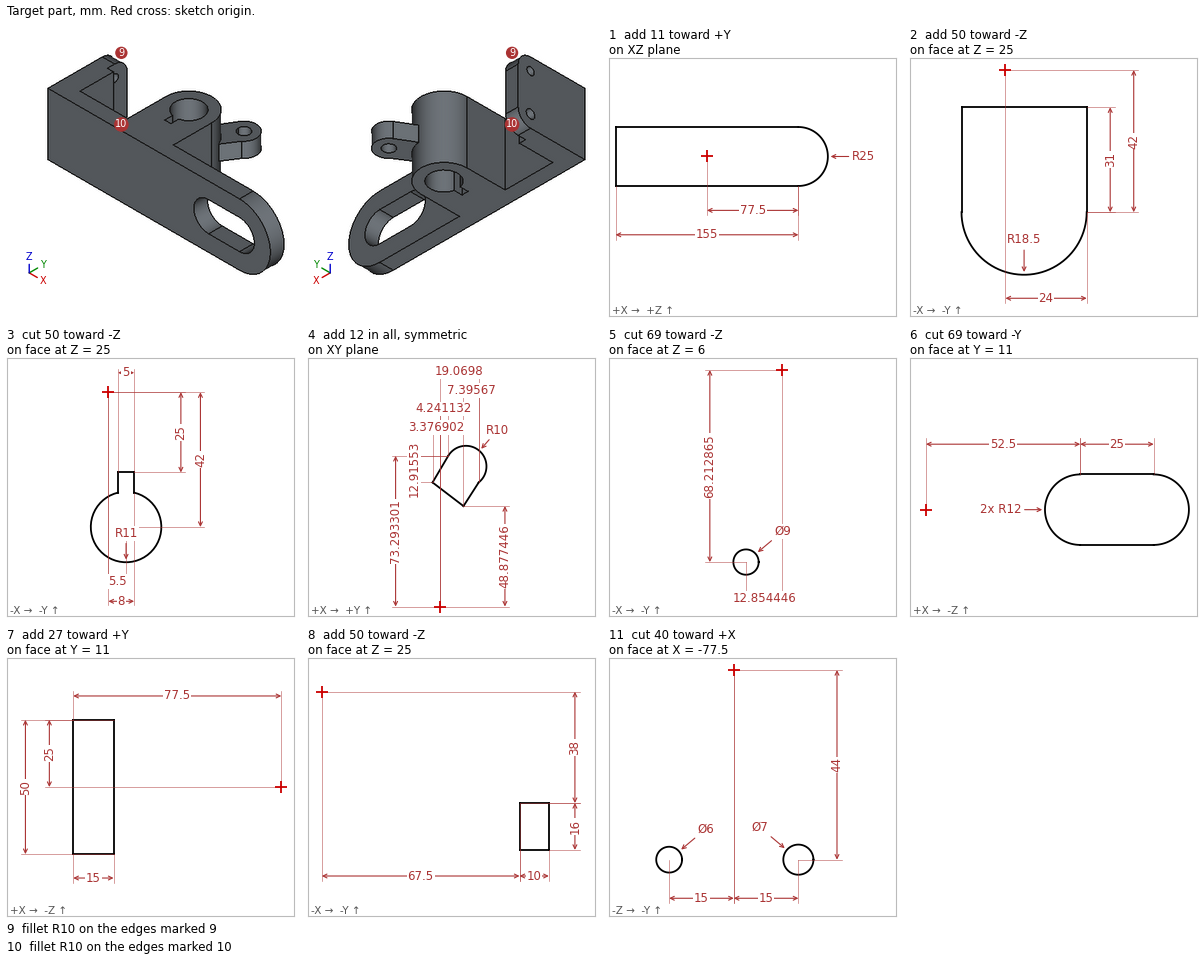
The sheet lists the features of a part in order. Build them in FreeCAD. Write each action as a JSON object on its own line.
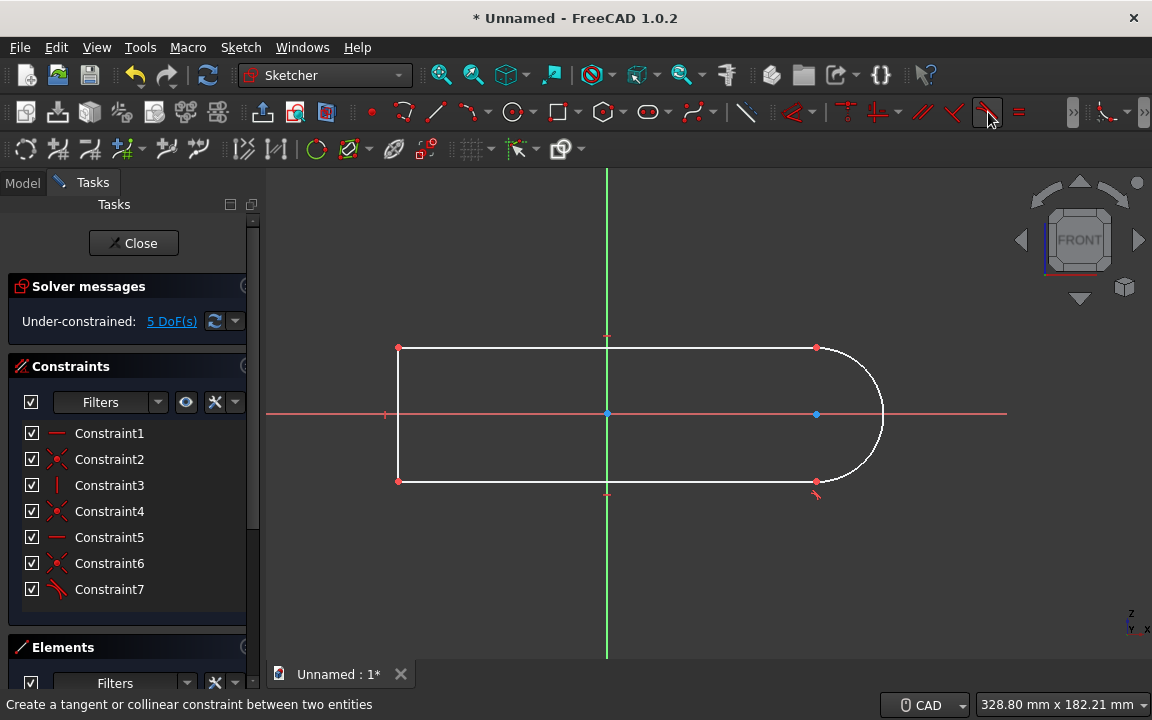
{"action": "left_click", "coordinate": [523, 348]}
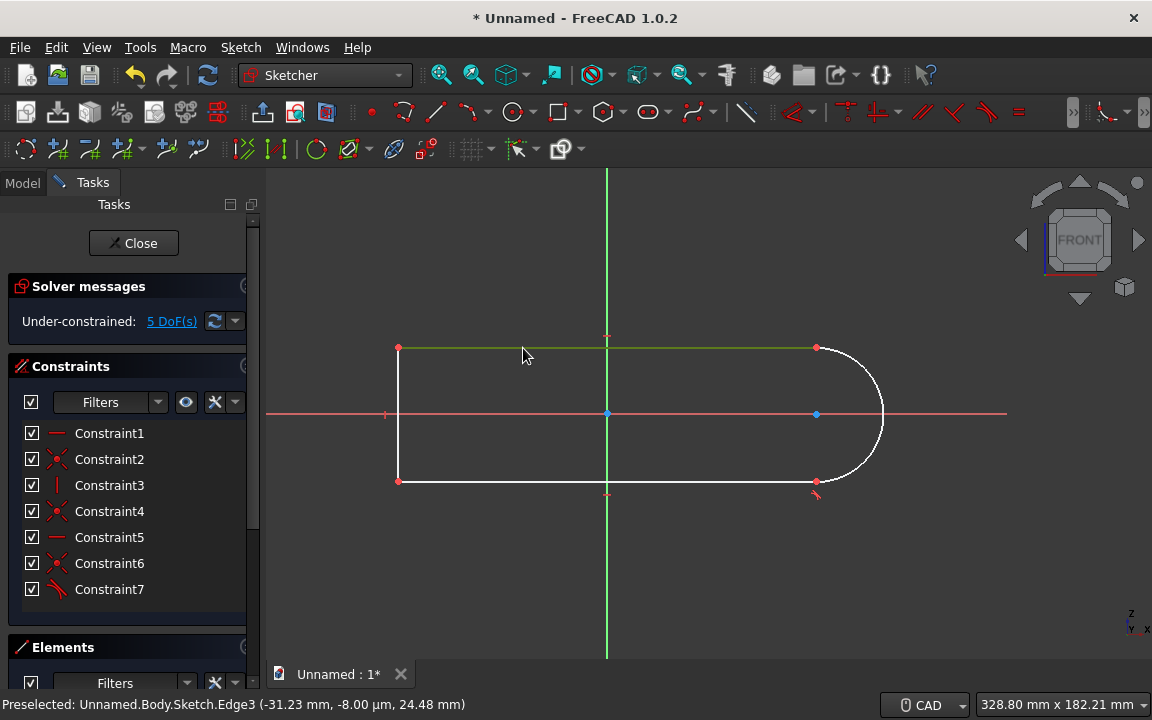
{"action": "left_click", "coordinate": [871, 454]}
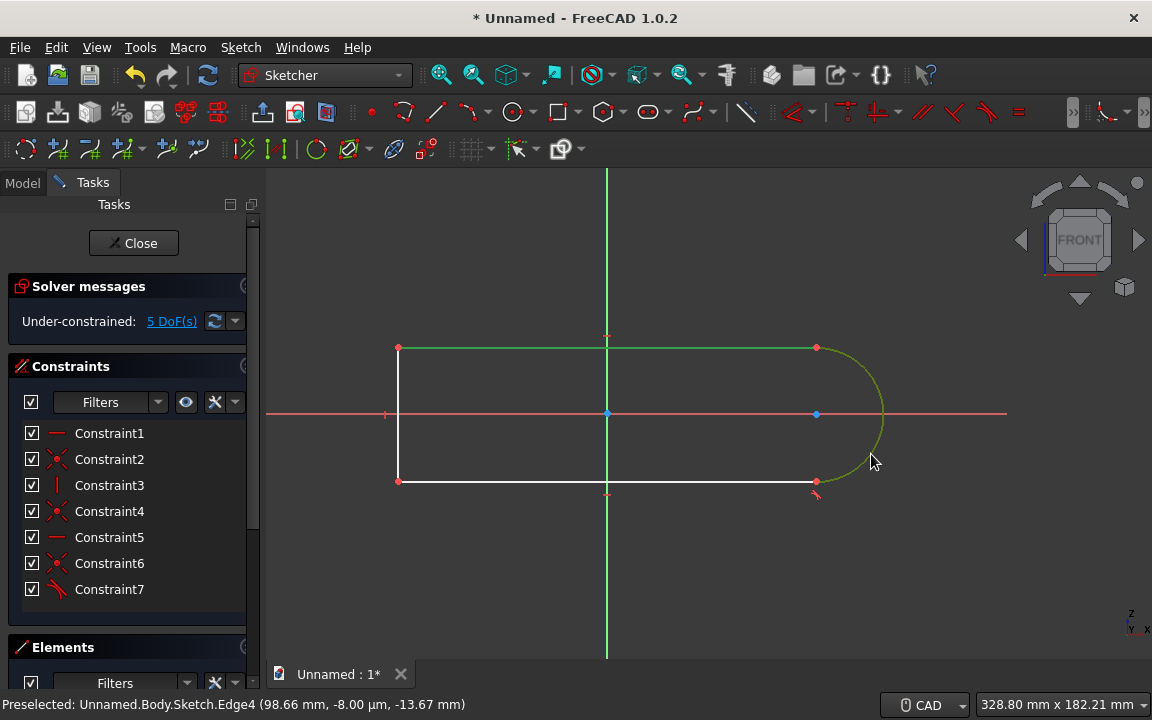
{"action": "left_click", "coordinate": [988, 112]}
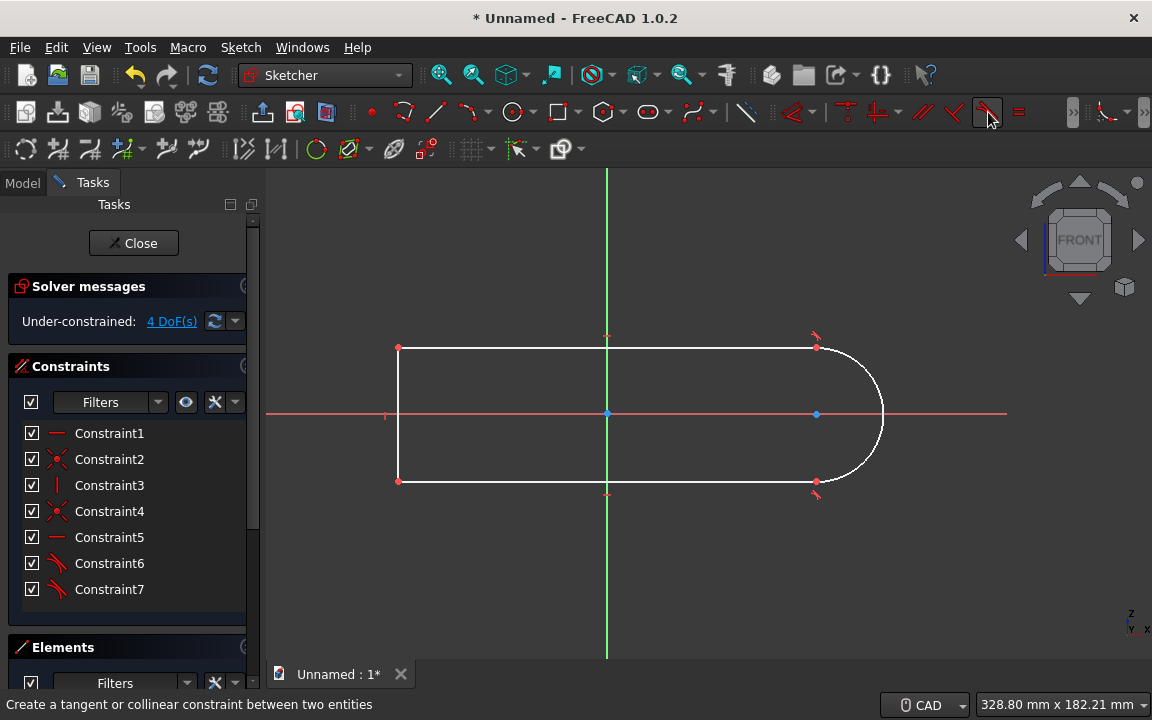
{"action": "left_click", "coordinate": [816, 415]}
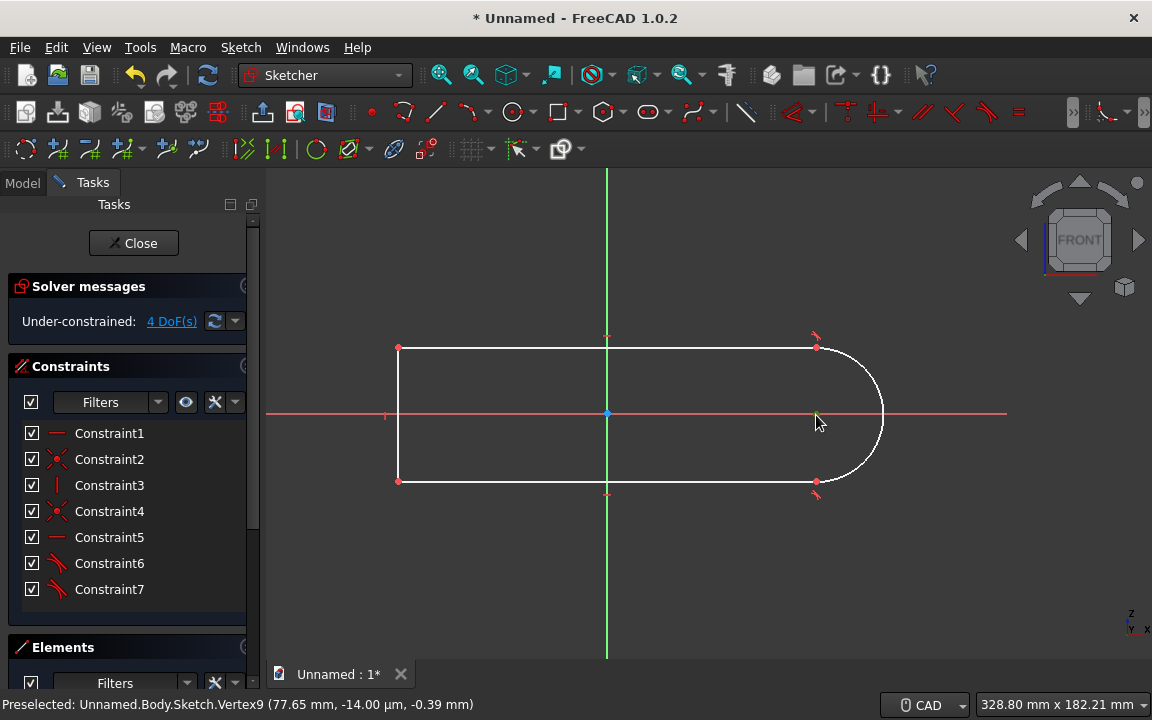
{"action": "left_click", "coordinate": [344, 414]}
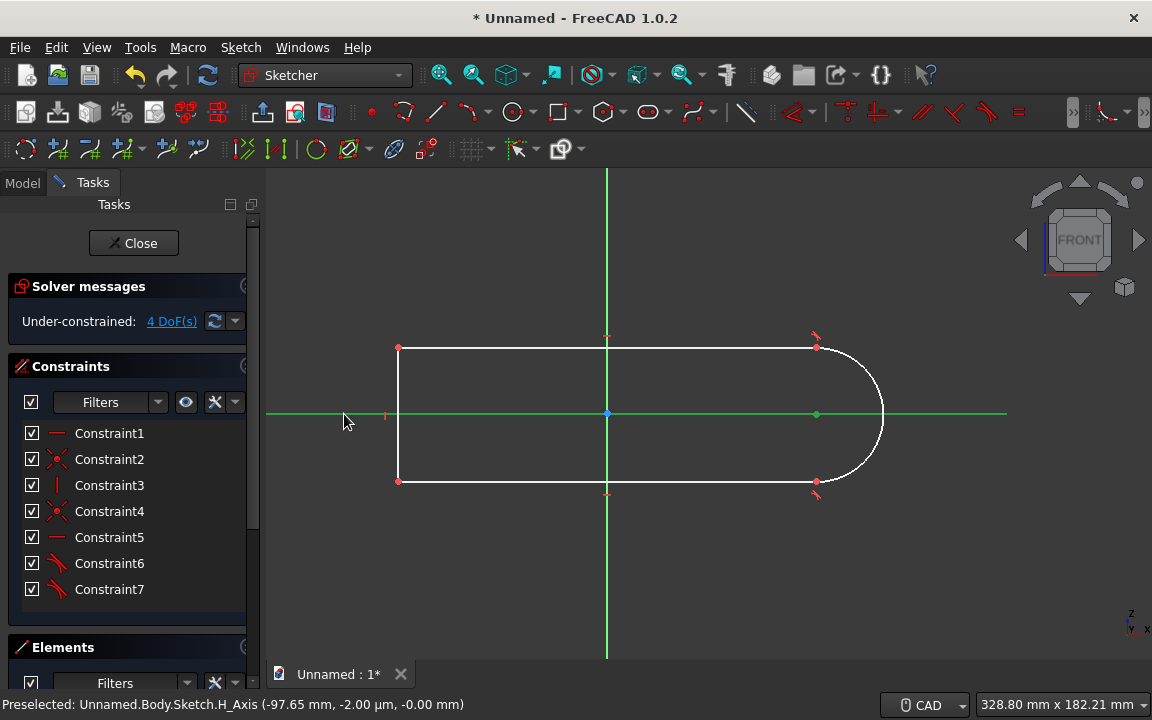
{"action": "left_click", "coordinate": [846, 112]}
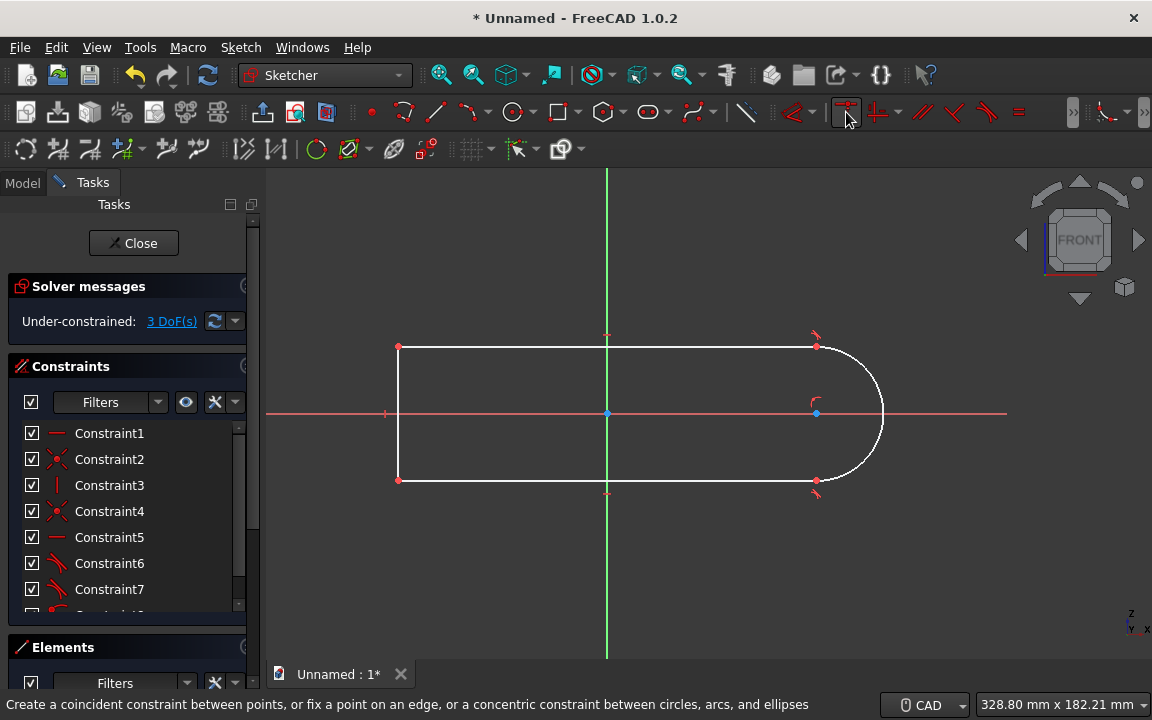
{"action": "left_click", "coordinate": [792, 112]}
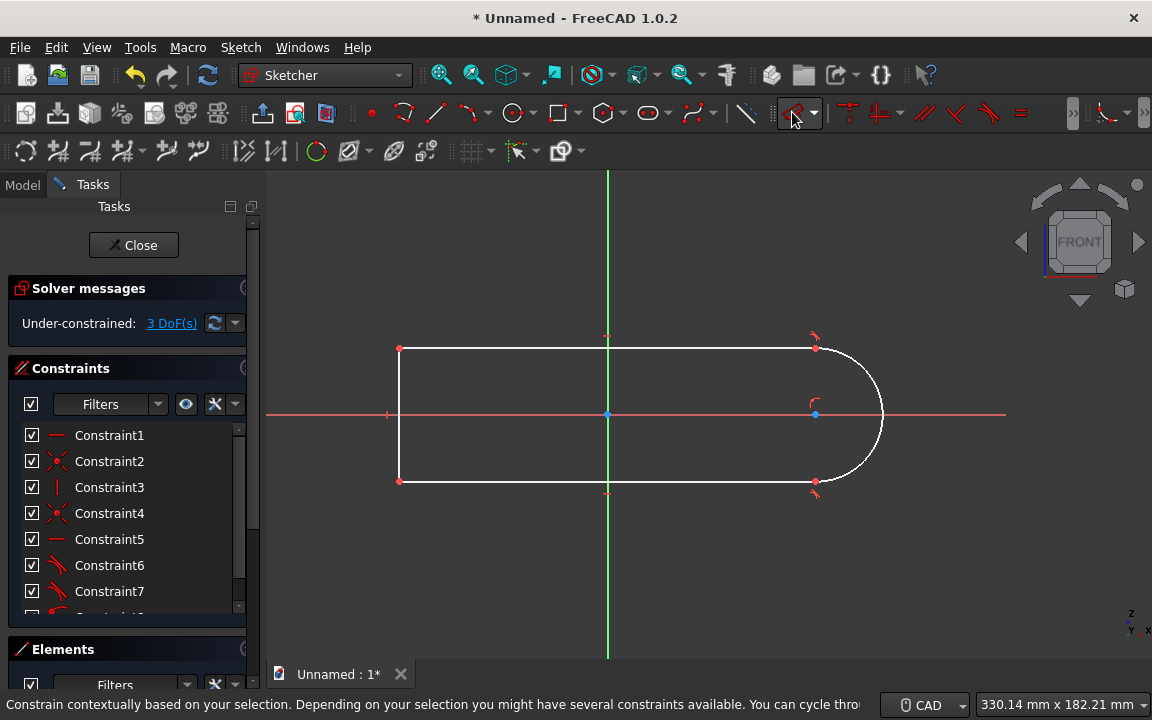
{"action": "left_click", "coordinate": [870, 454]}
{"action": "left_click", "coordinate": [896, 473]}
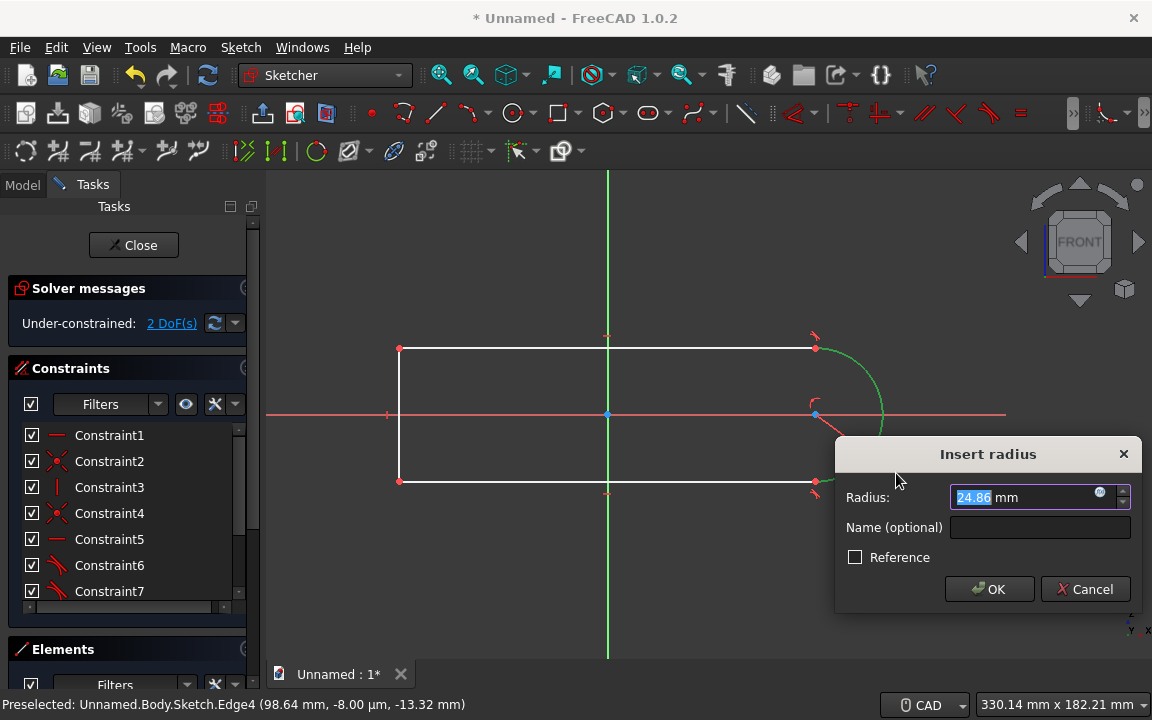
{"action": "type", "text": "25"}
{"action": "key", "text": "Return"}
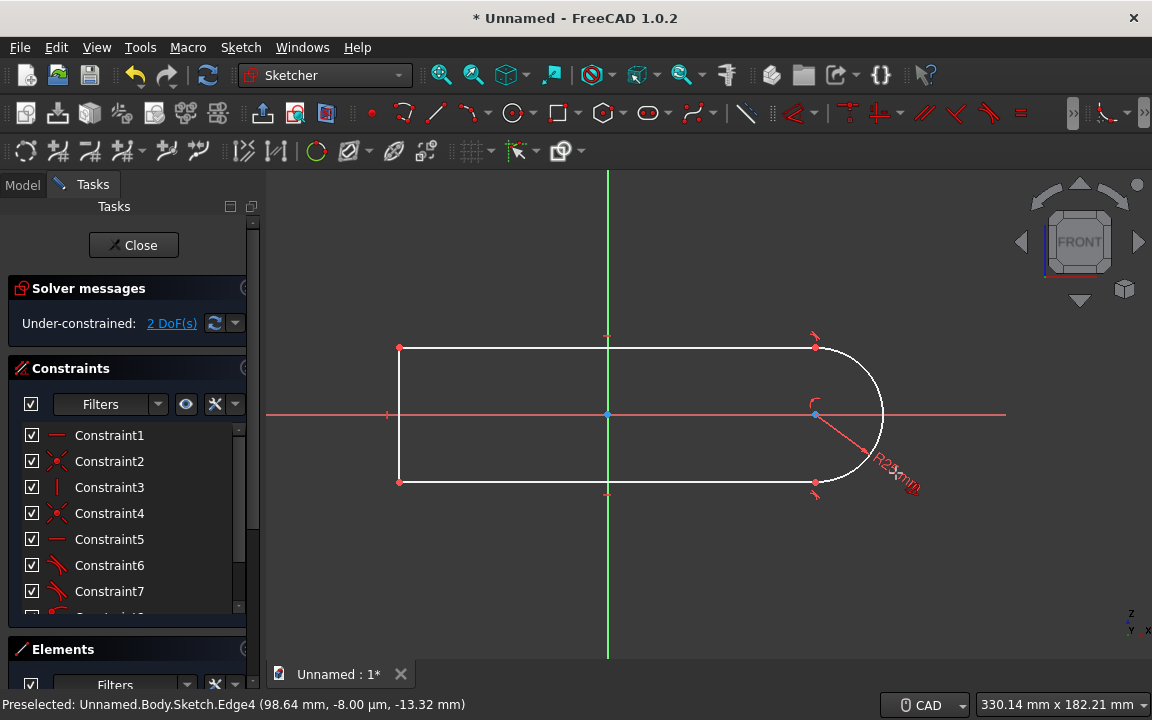
{"action": "left_click", "coordinate": [691, 482]}
{"action": "left_click", "coordinate": [512, 516]}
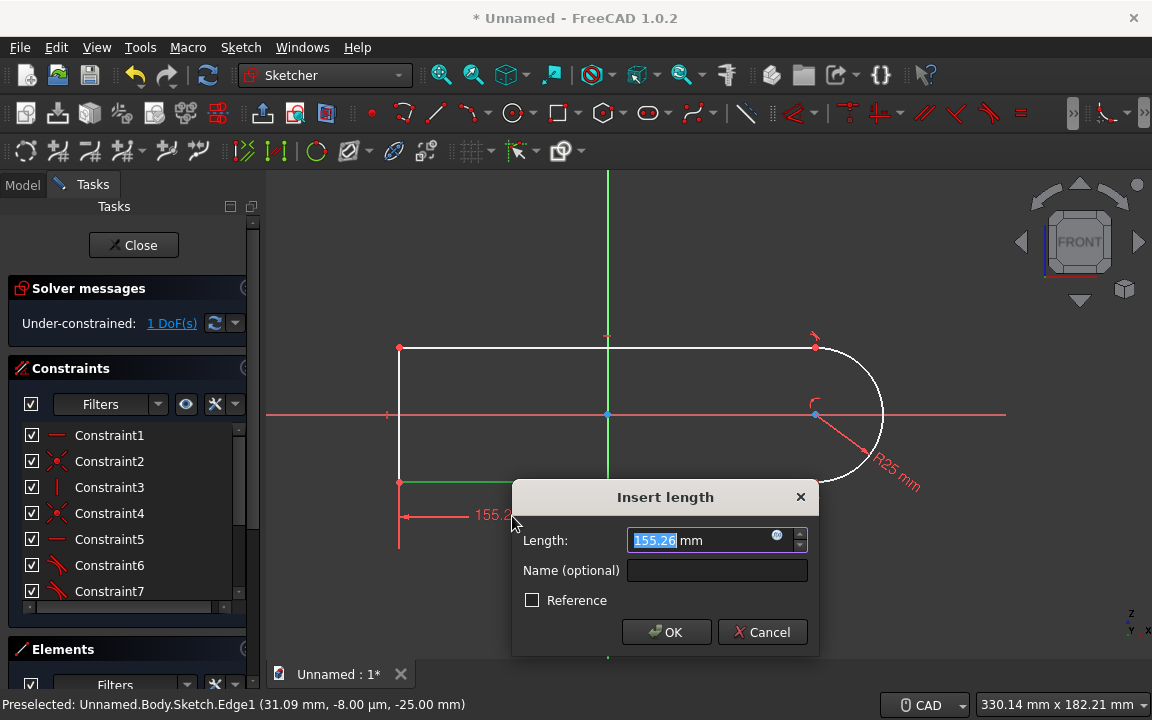
{"action": "type", "text": "155"}
{"action": "key", "text": "Return"}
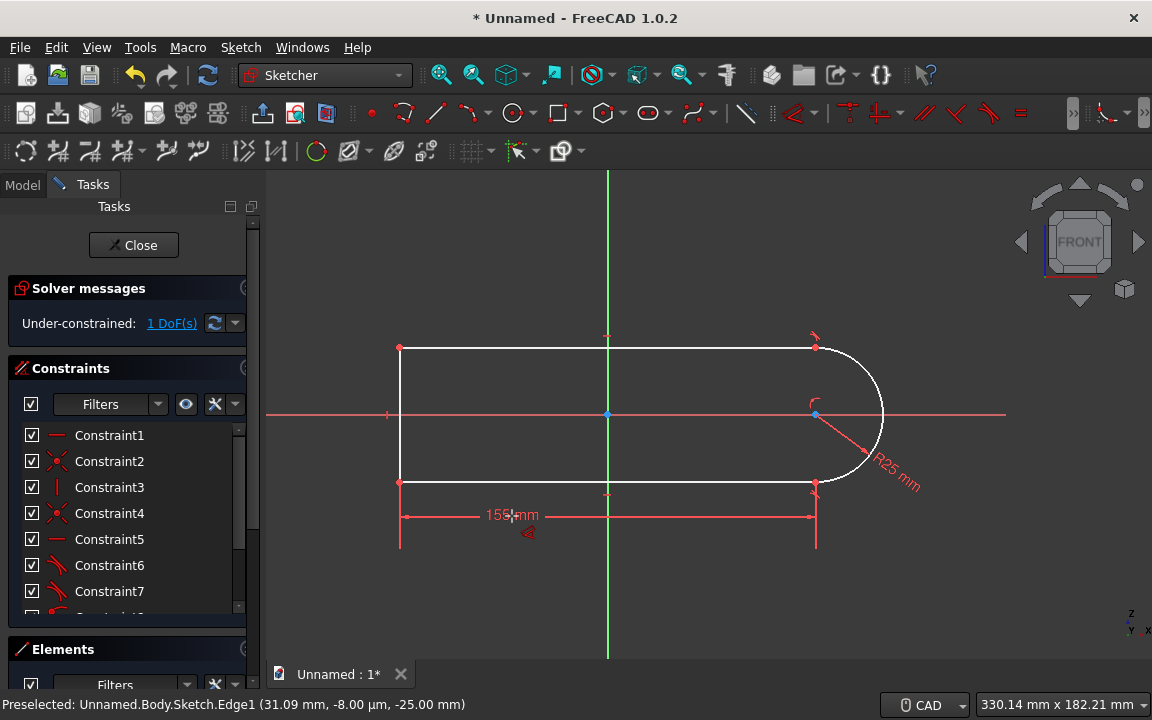
{"action": "left_click", "coordinate": [816, 482]}
{"action": "left_click", "coordinate": [712, 516]}